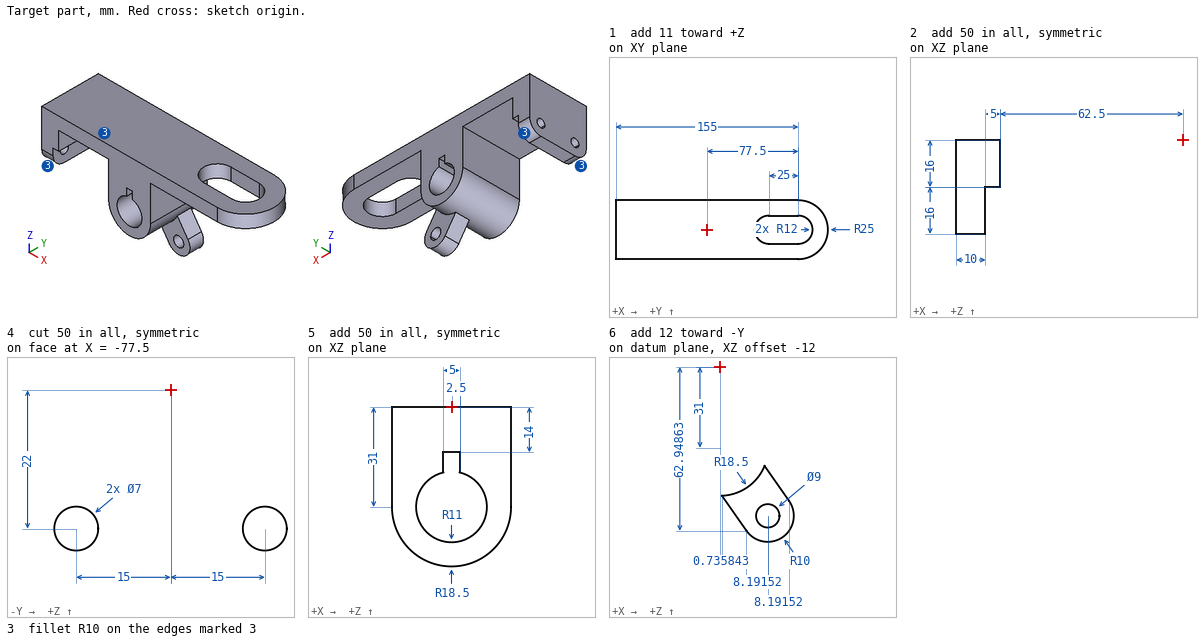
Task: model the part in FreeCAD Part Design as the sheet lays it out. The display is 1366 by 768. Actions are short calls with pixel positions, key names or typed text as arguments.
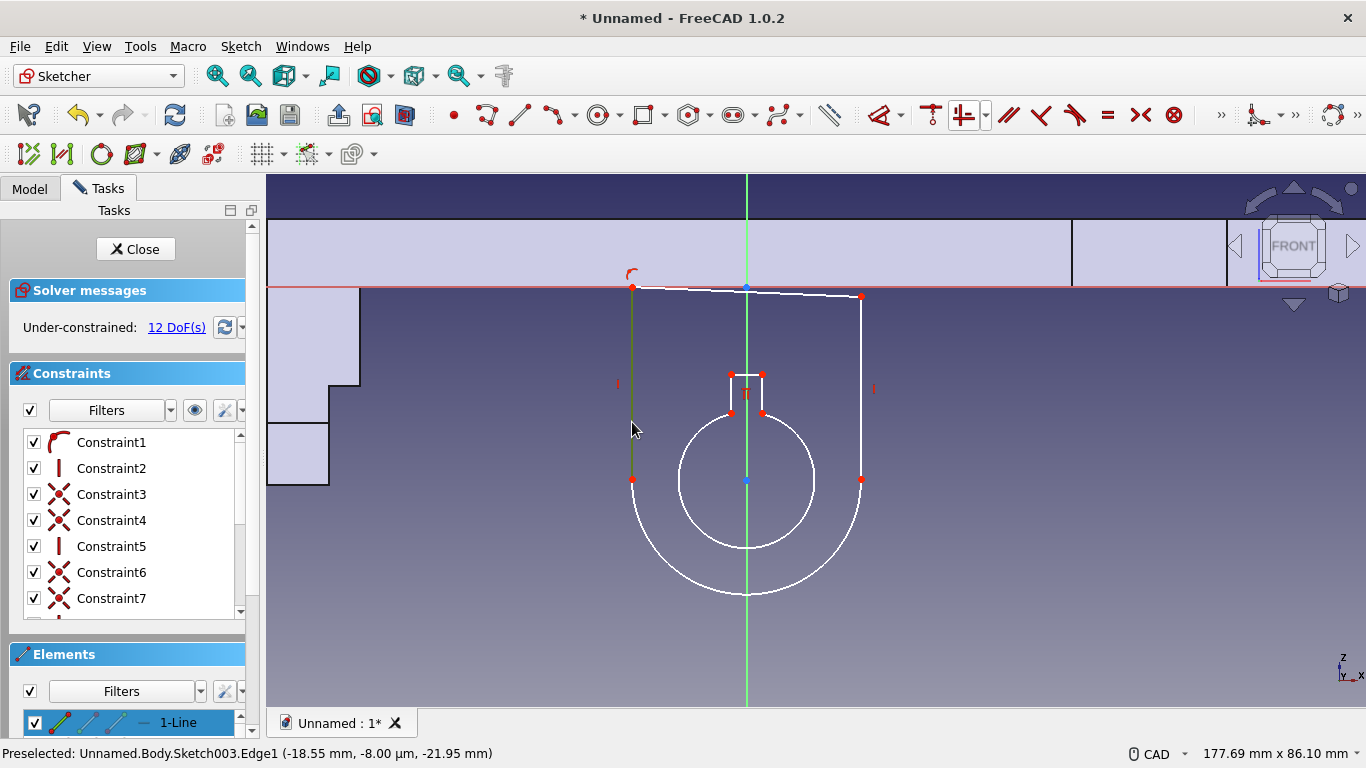
click(679, 573)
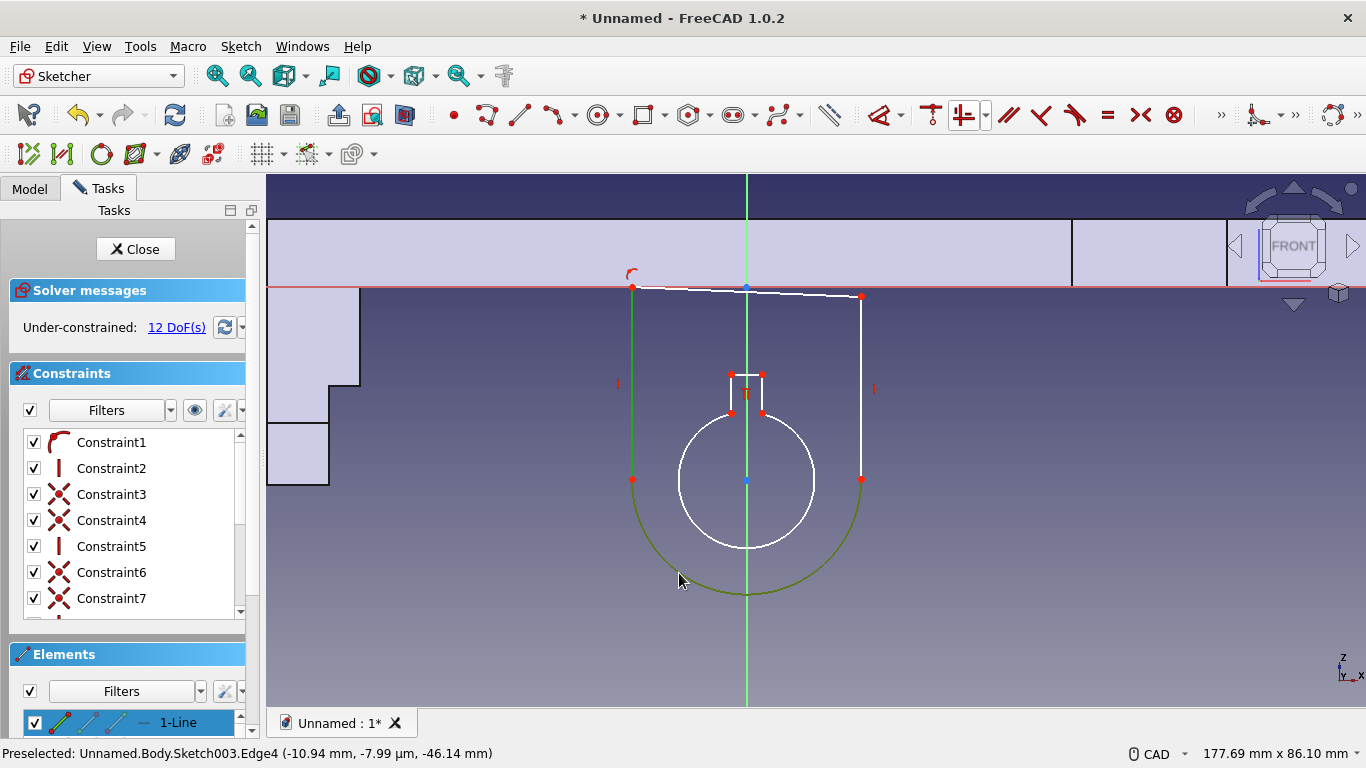
click(1075, 116)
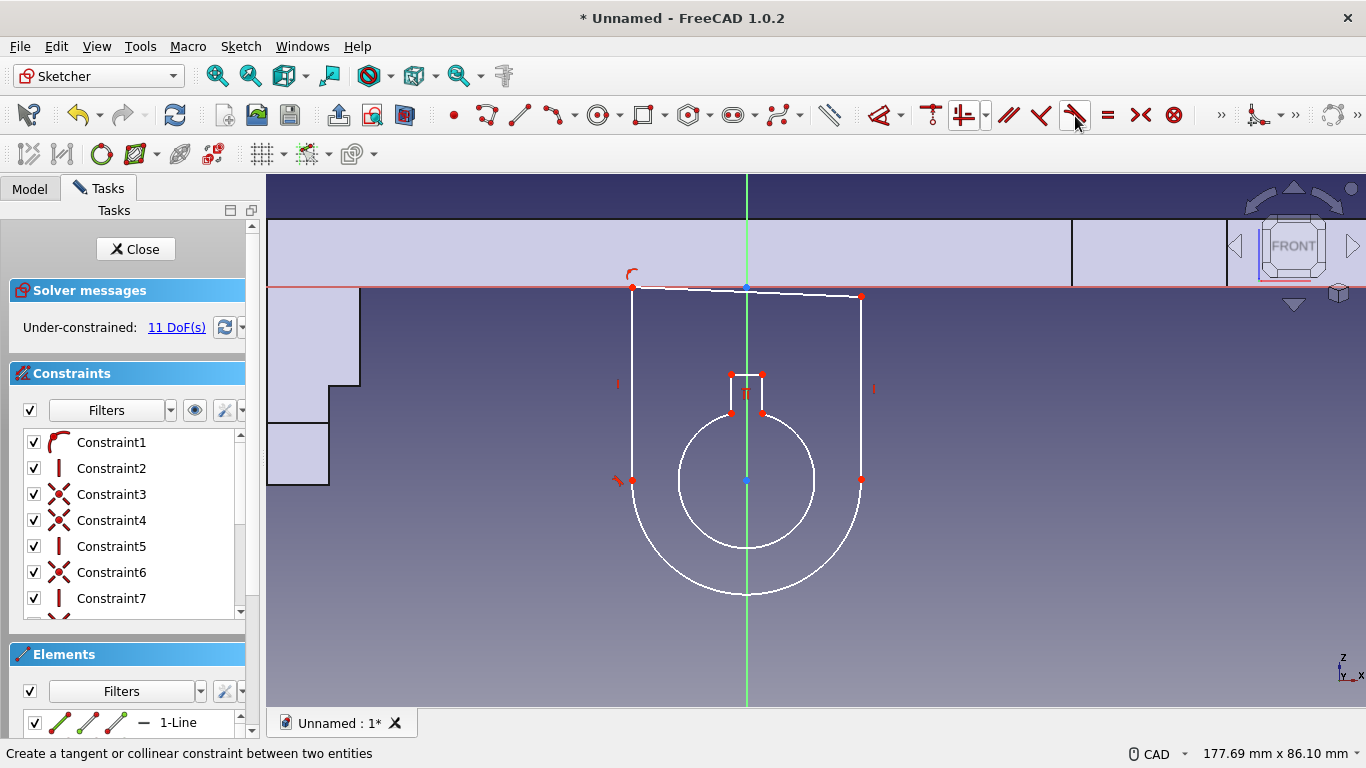
click(861, 352)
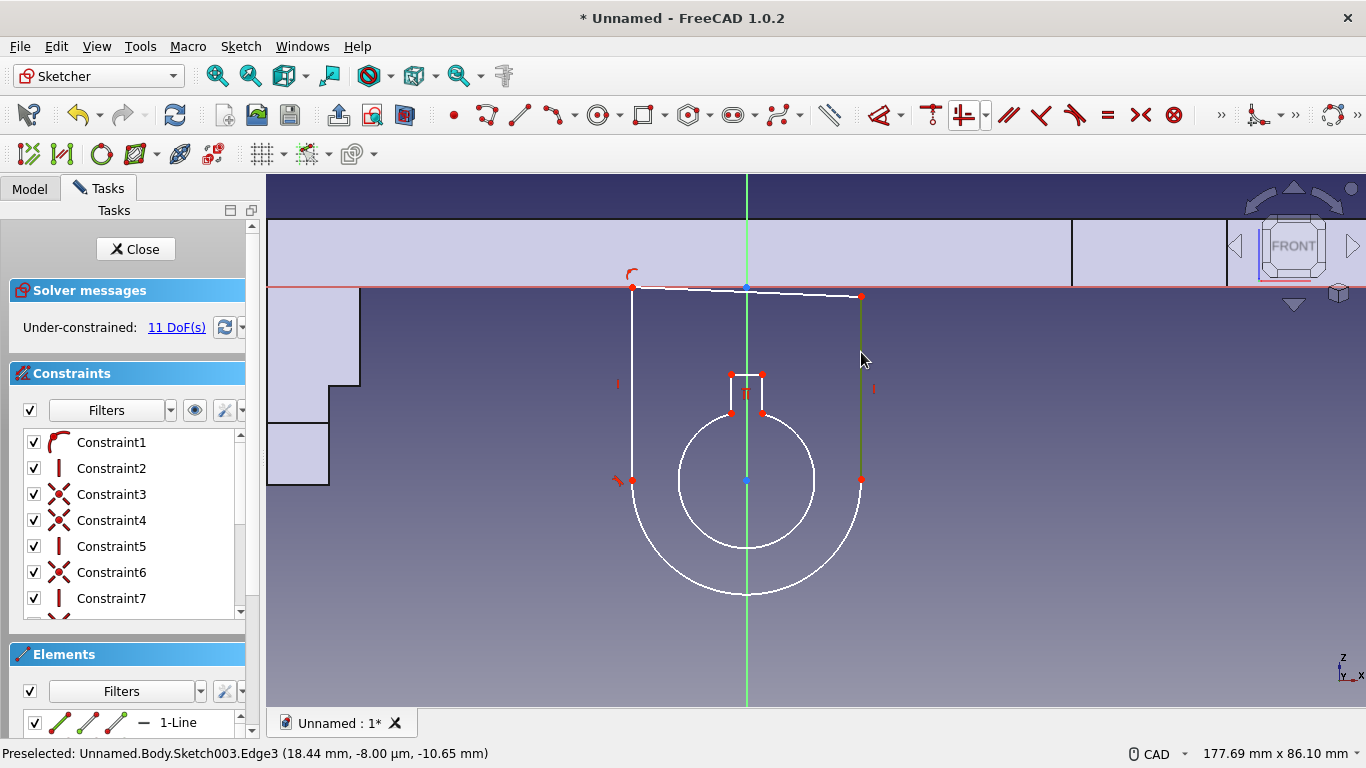
click(679, 573)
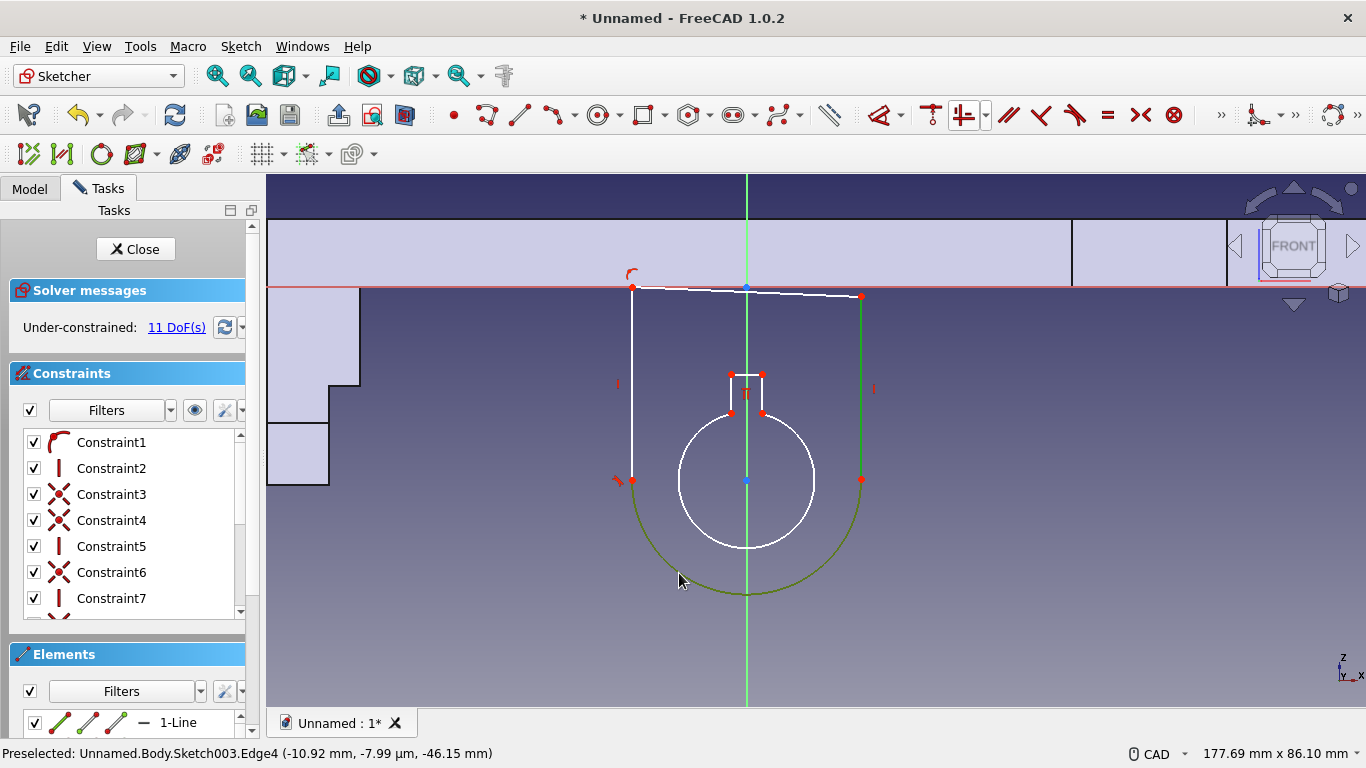
key(t)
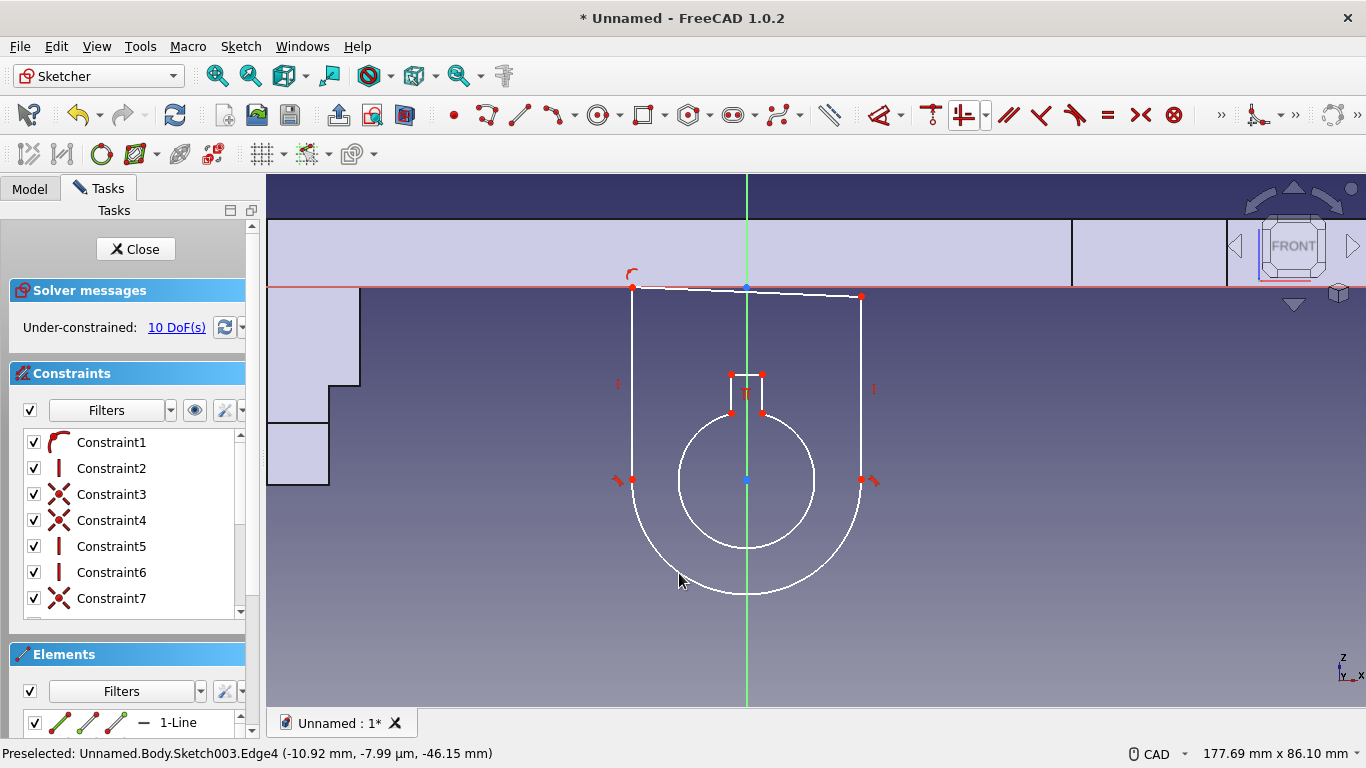
click(701, 290)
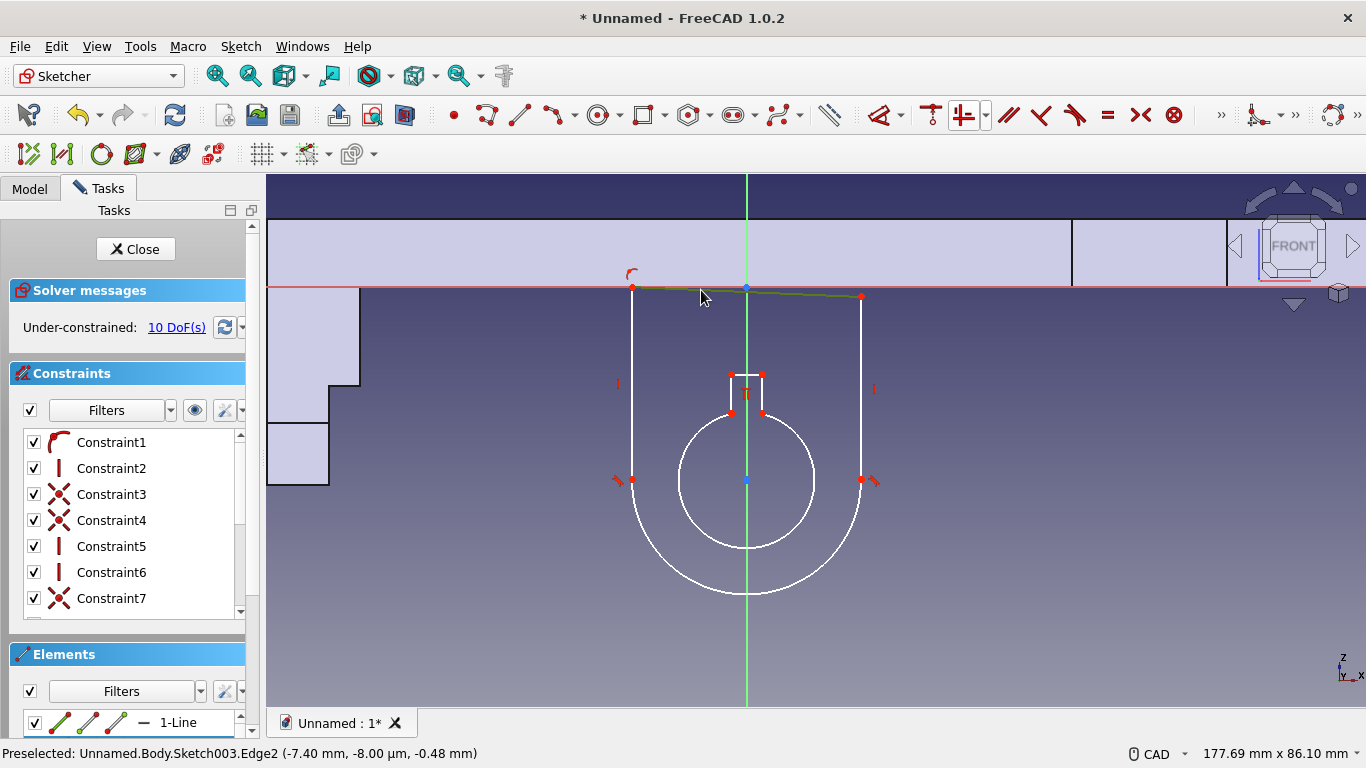
key(h)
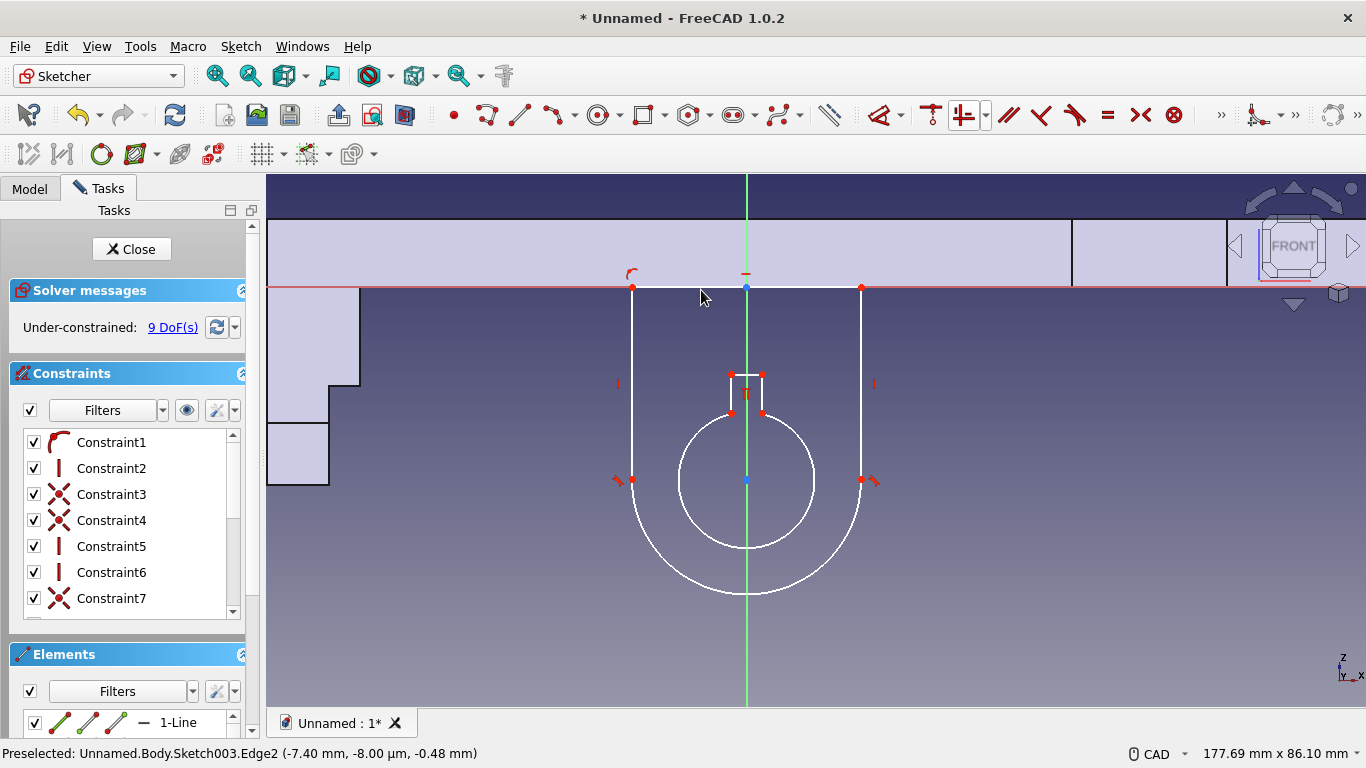
click(679, 573)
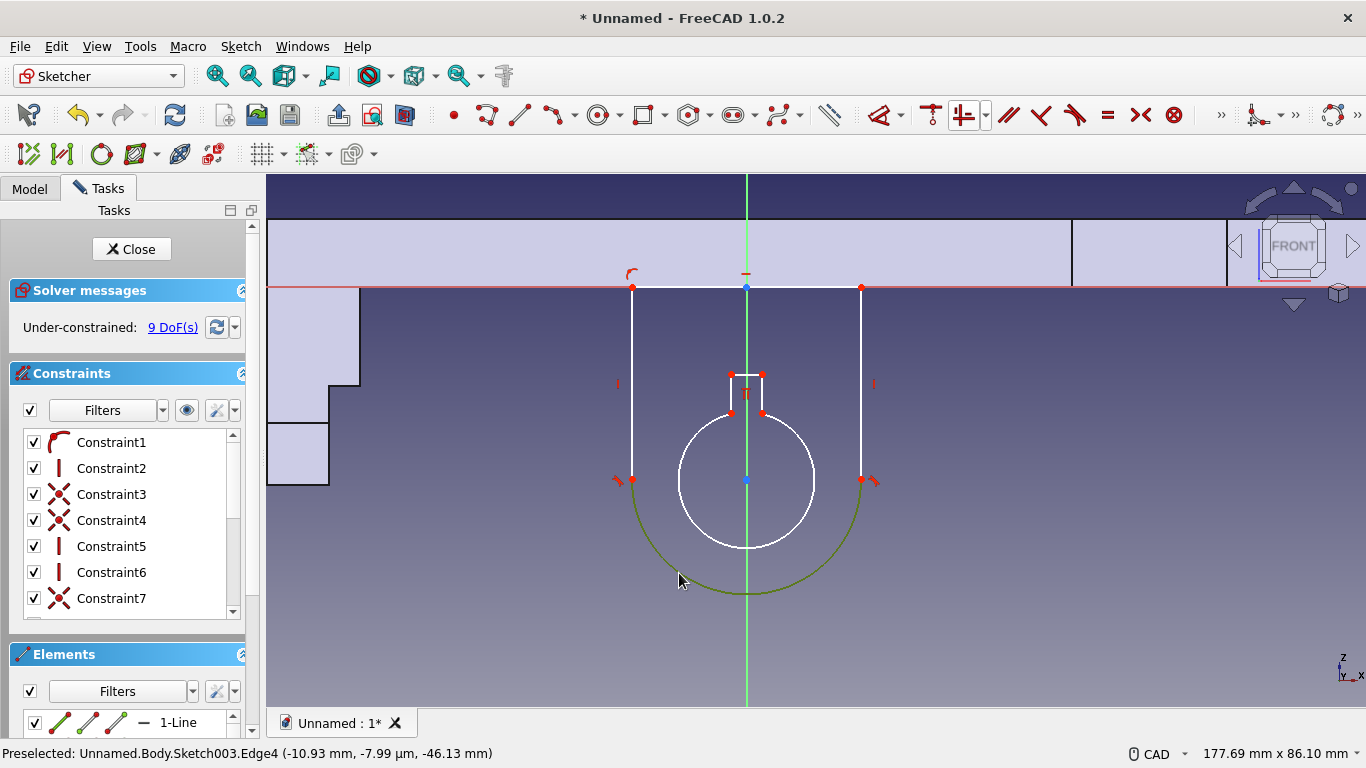
click(684, 507)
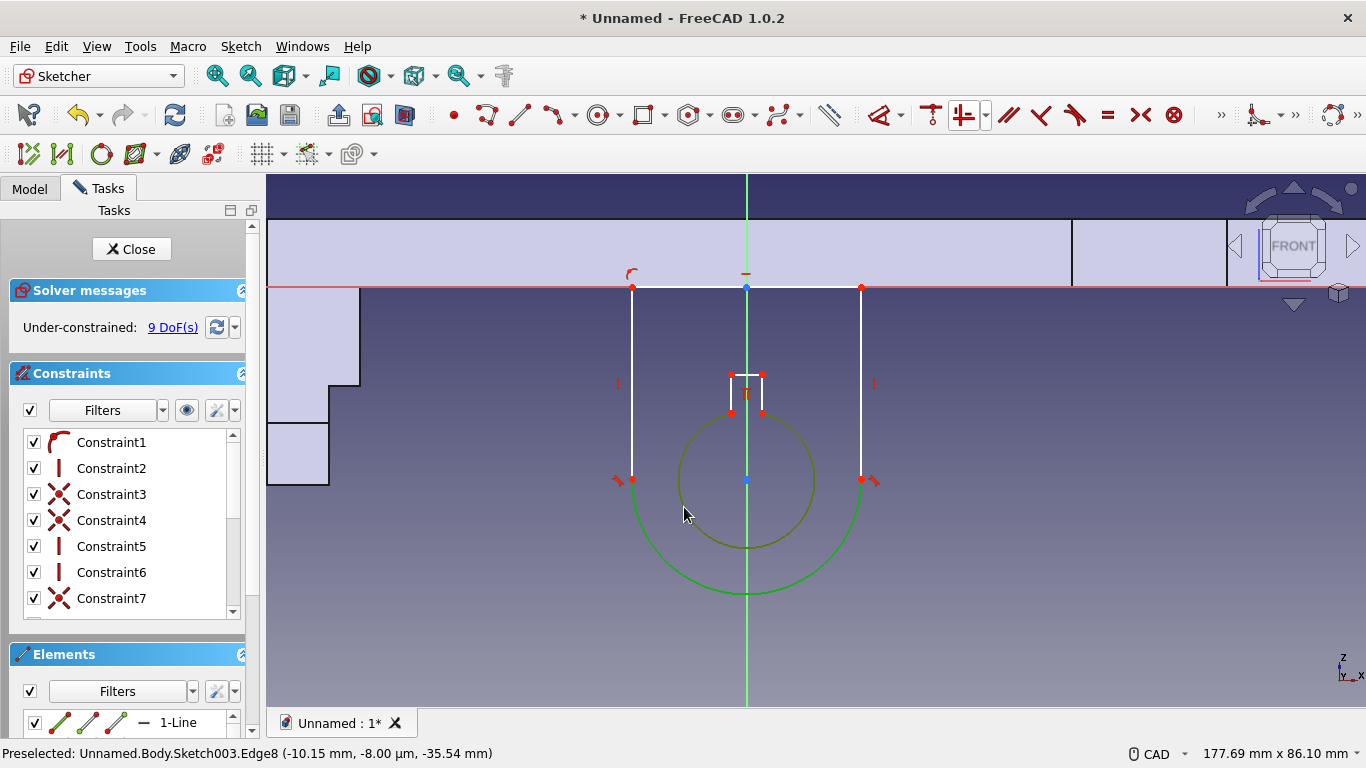
click(931, 116)